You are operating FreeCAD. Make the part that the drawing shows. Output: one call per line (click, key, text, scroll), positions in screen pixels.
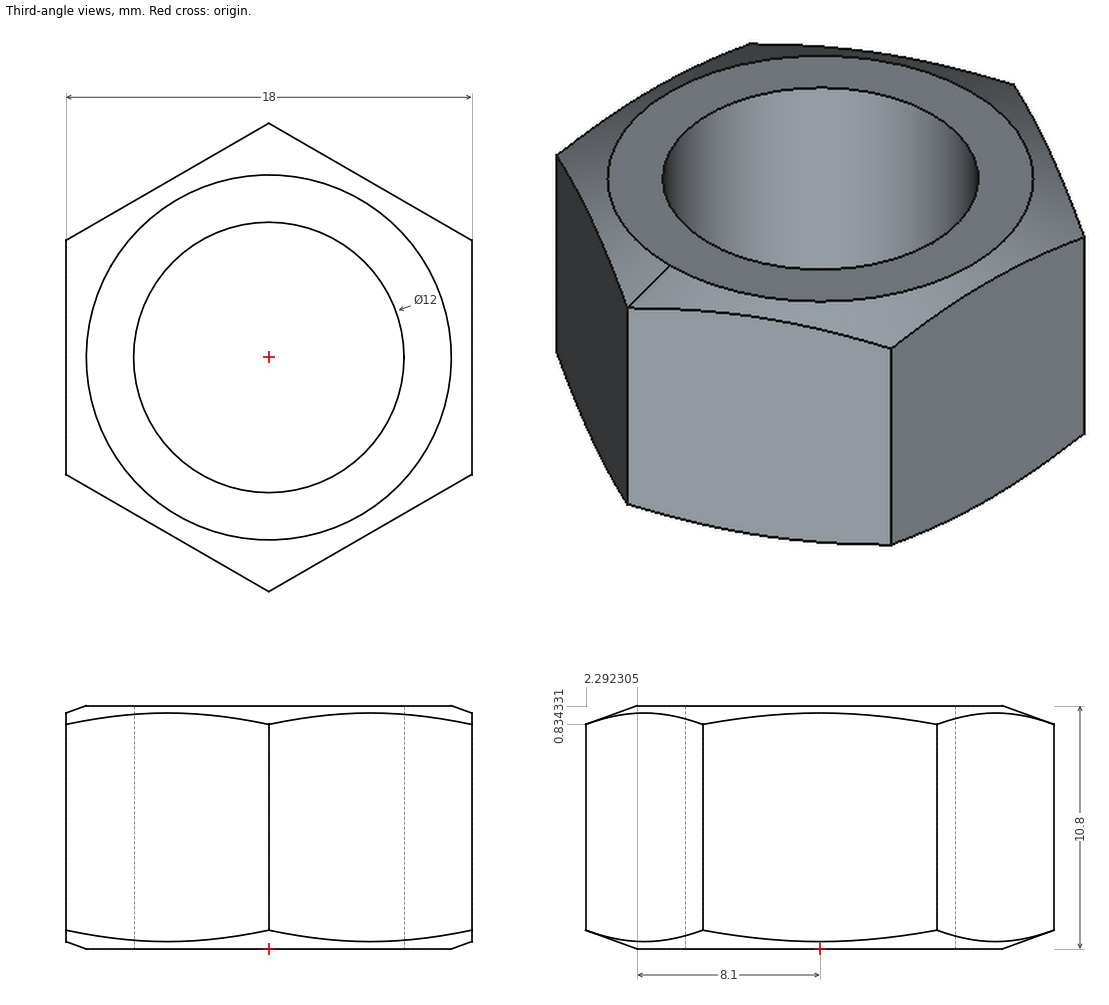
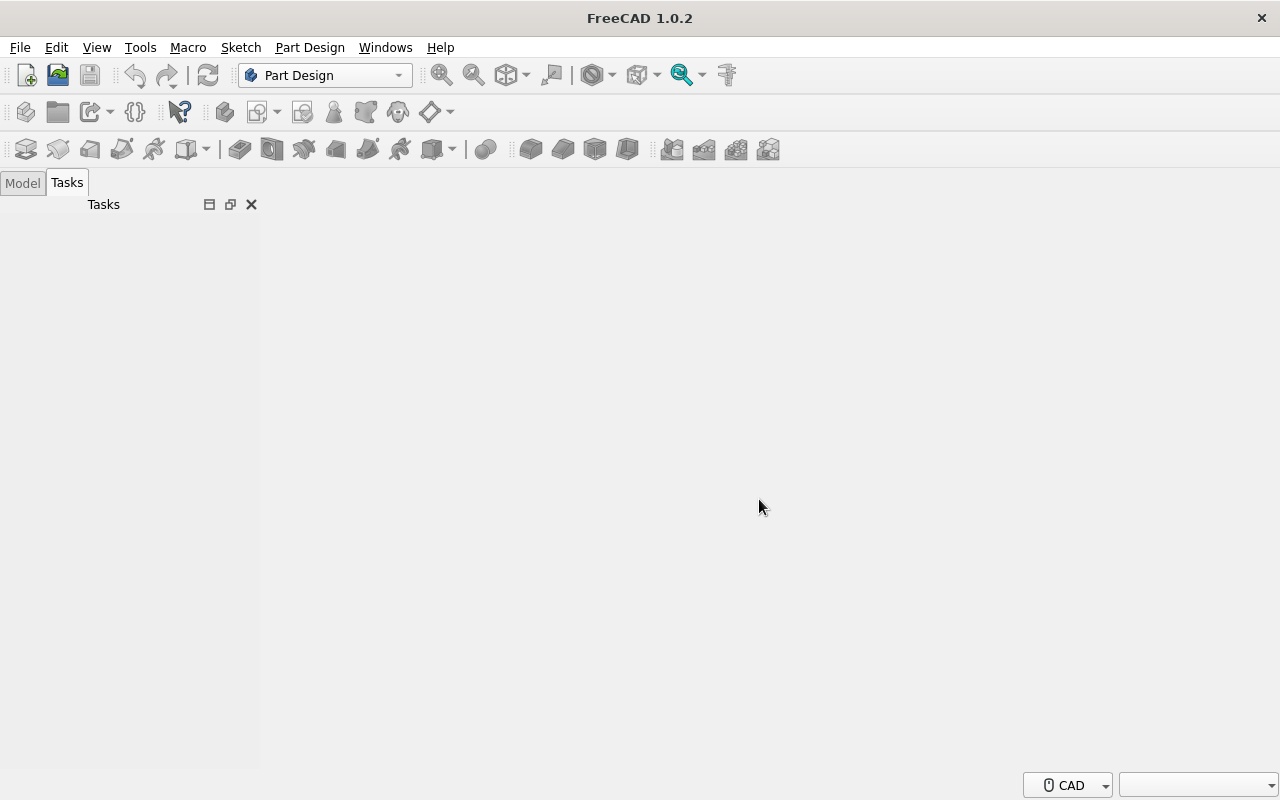
key(ctrl+n)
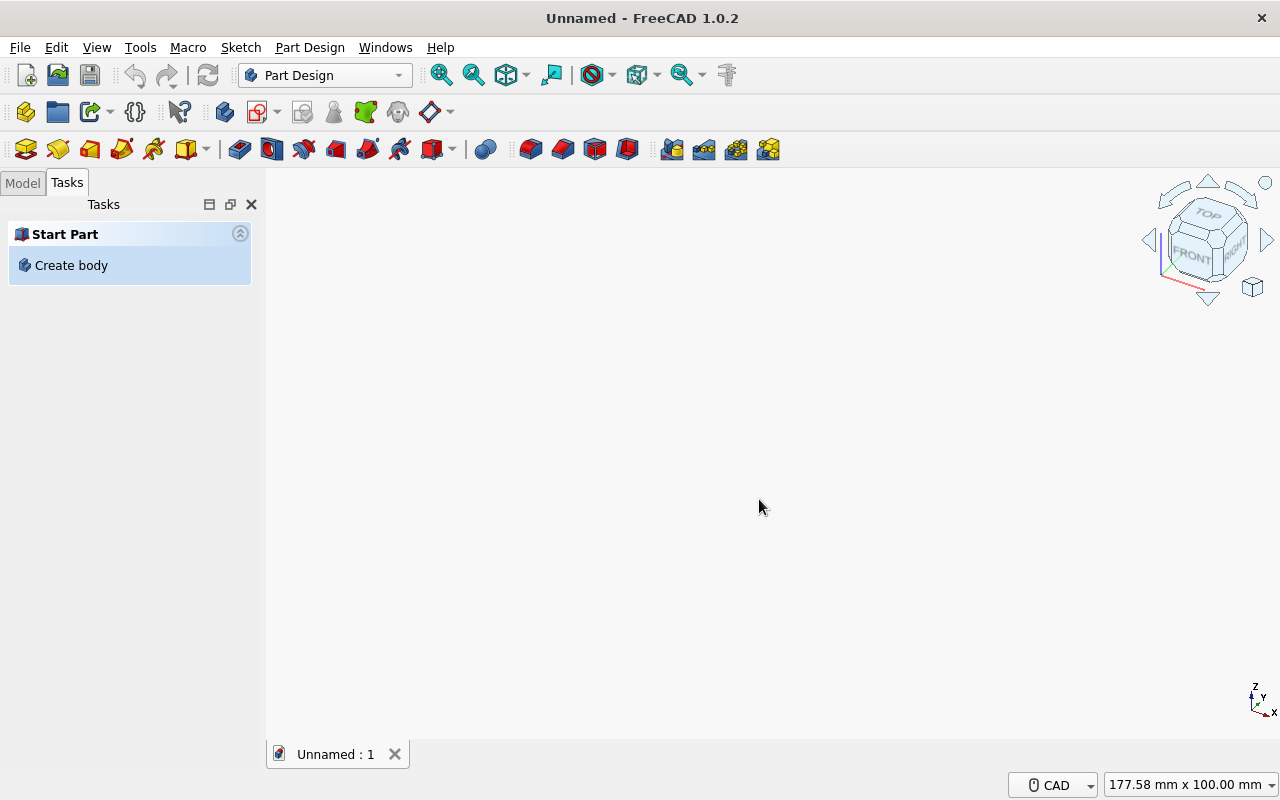
click(258, 112)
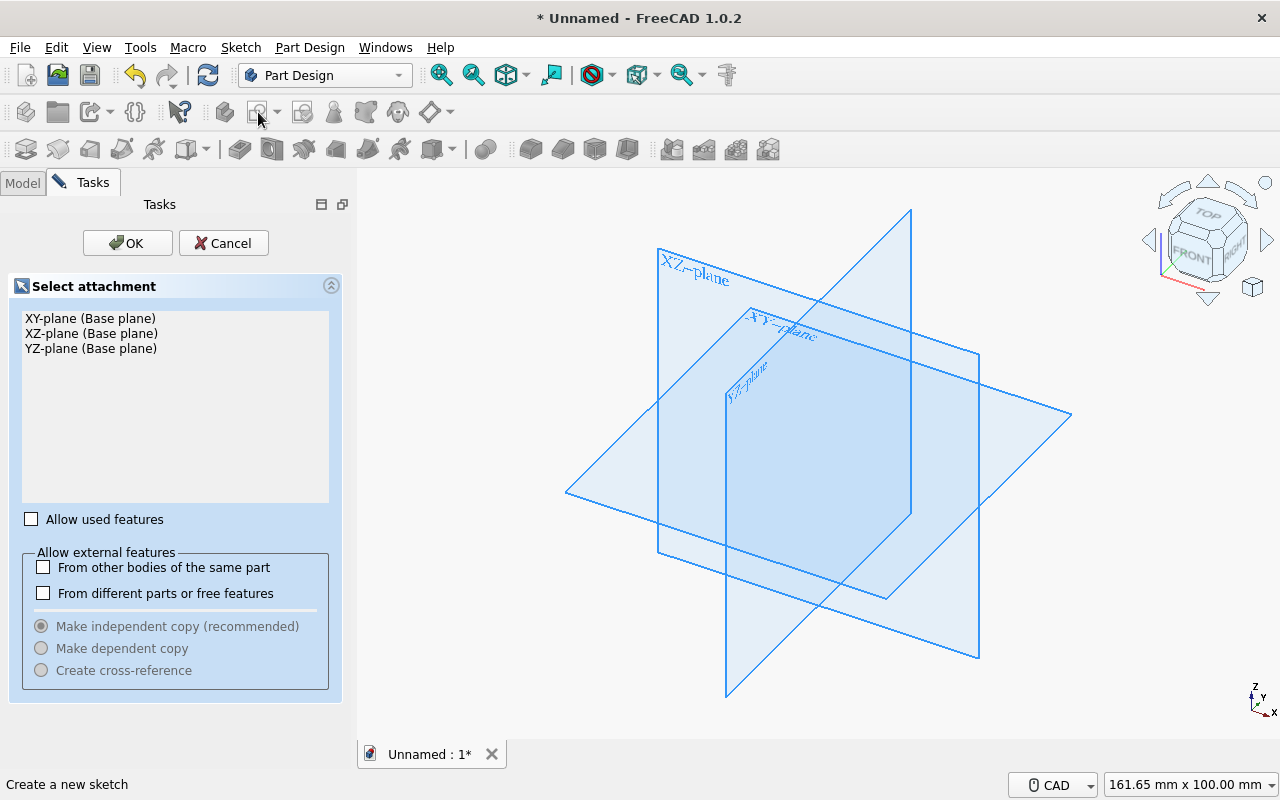
click(82, 318)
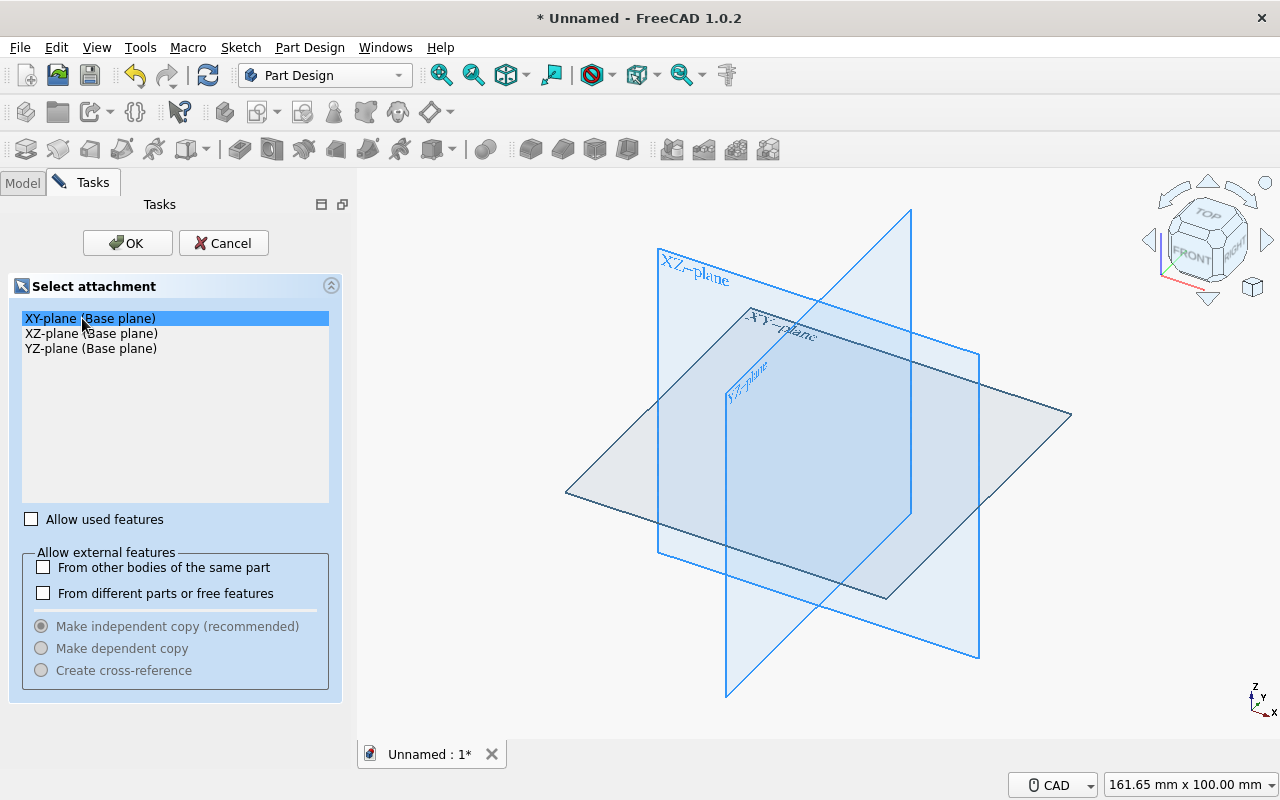
click(128, 243)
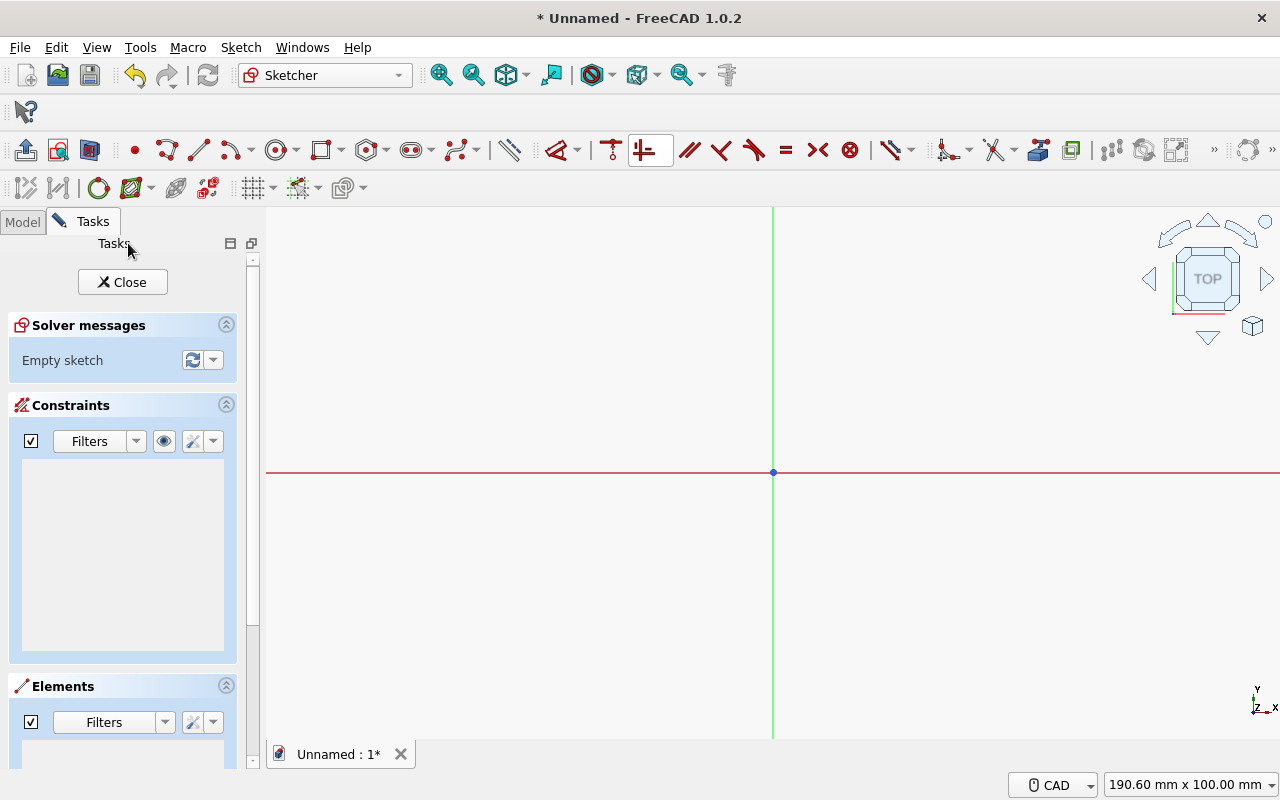
scroll(803, 473, up, 6)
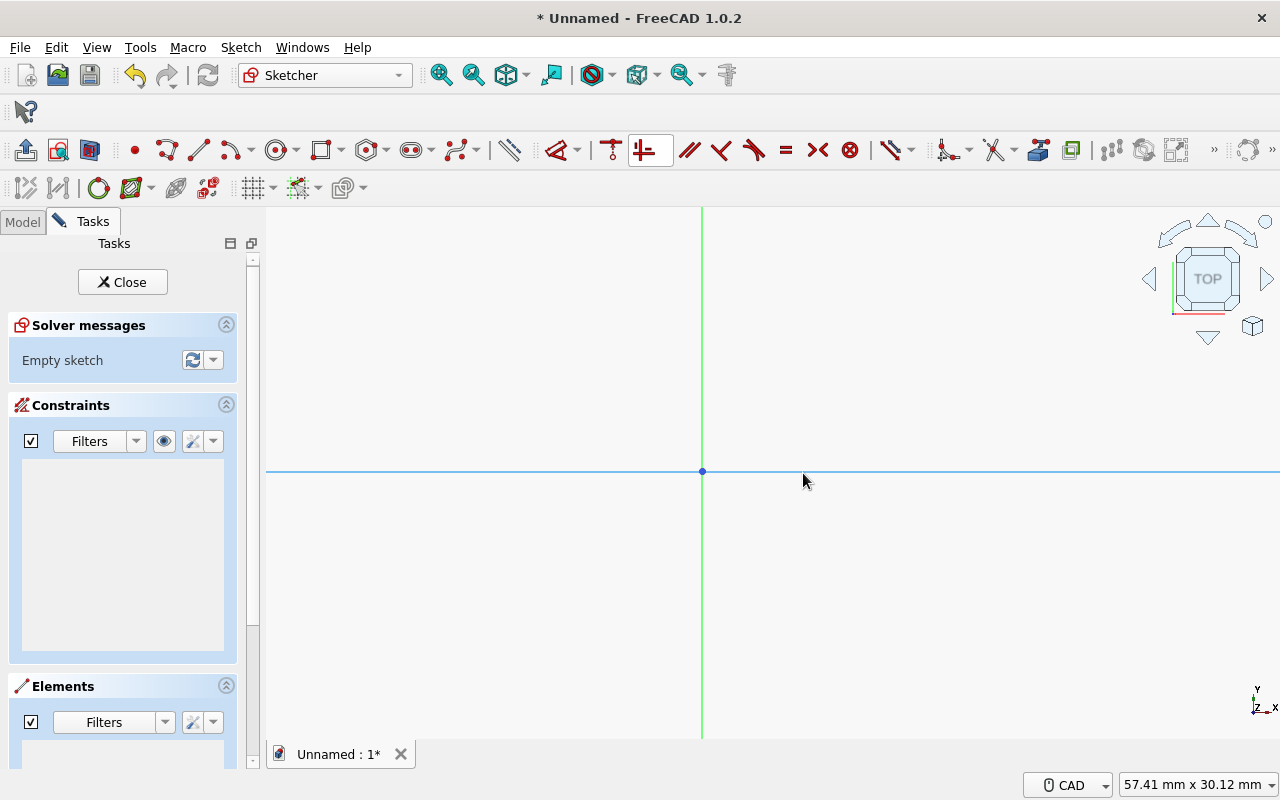
click(366, 150)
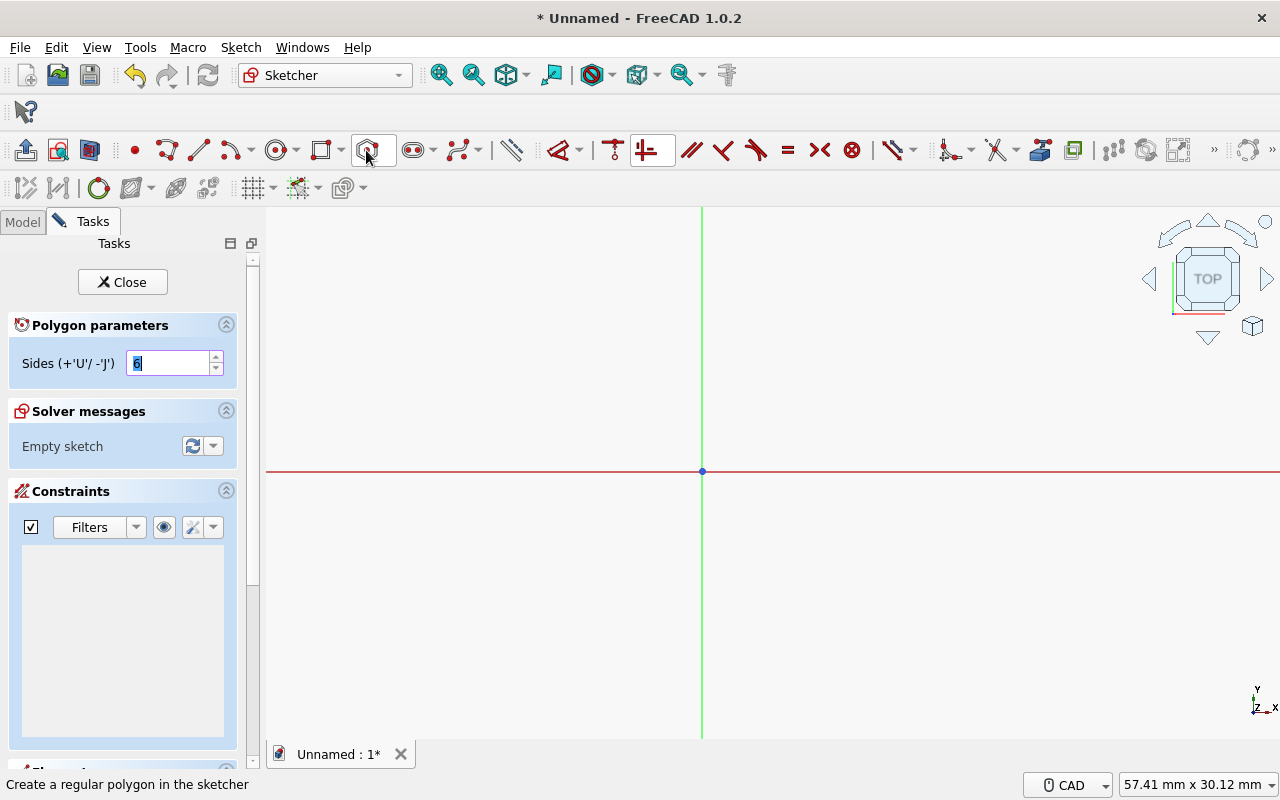
click(702, 472)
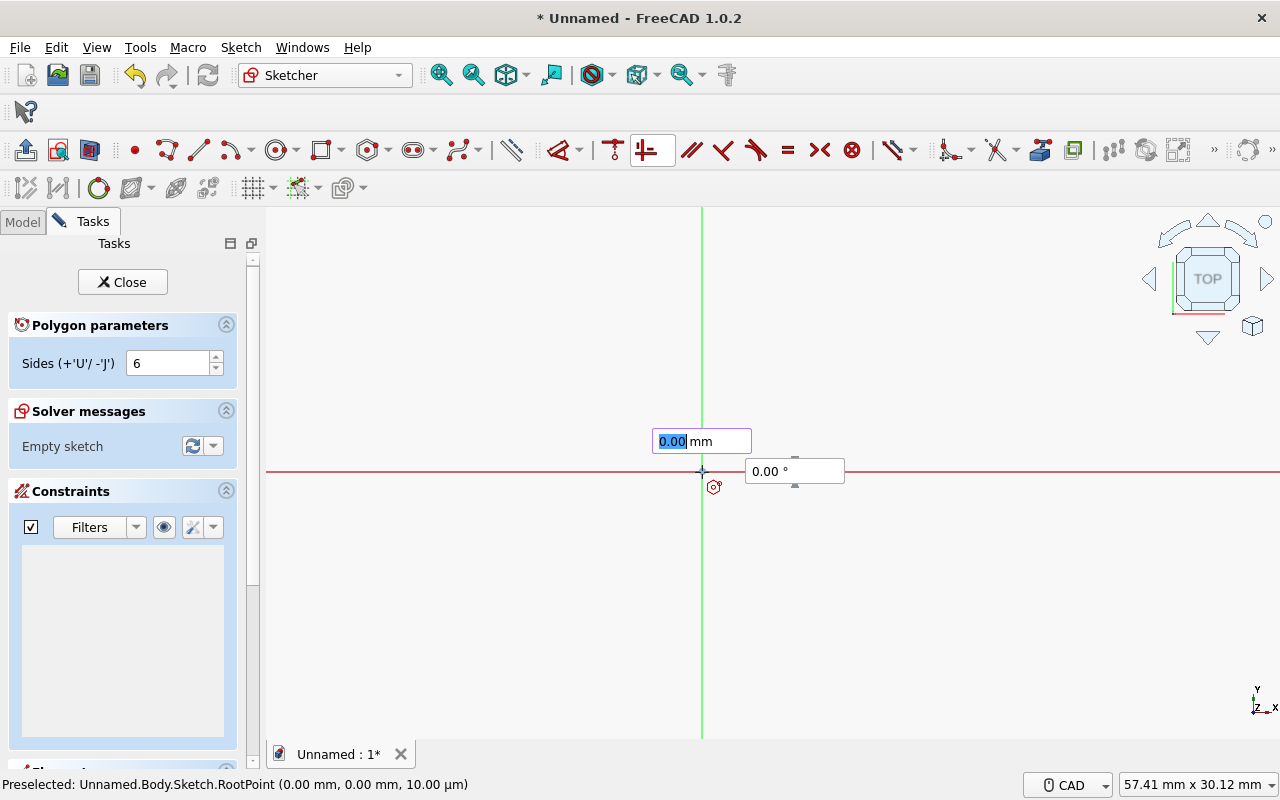
click(702, 288)
right_click(702, 288)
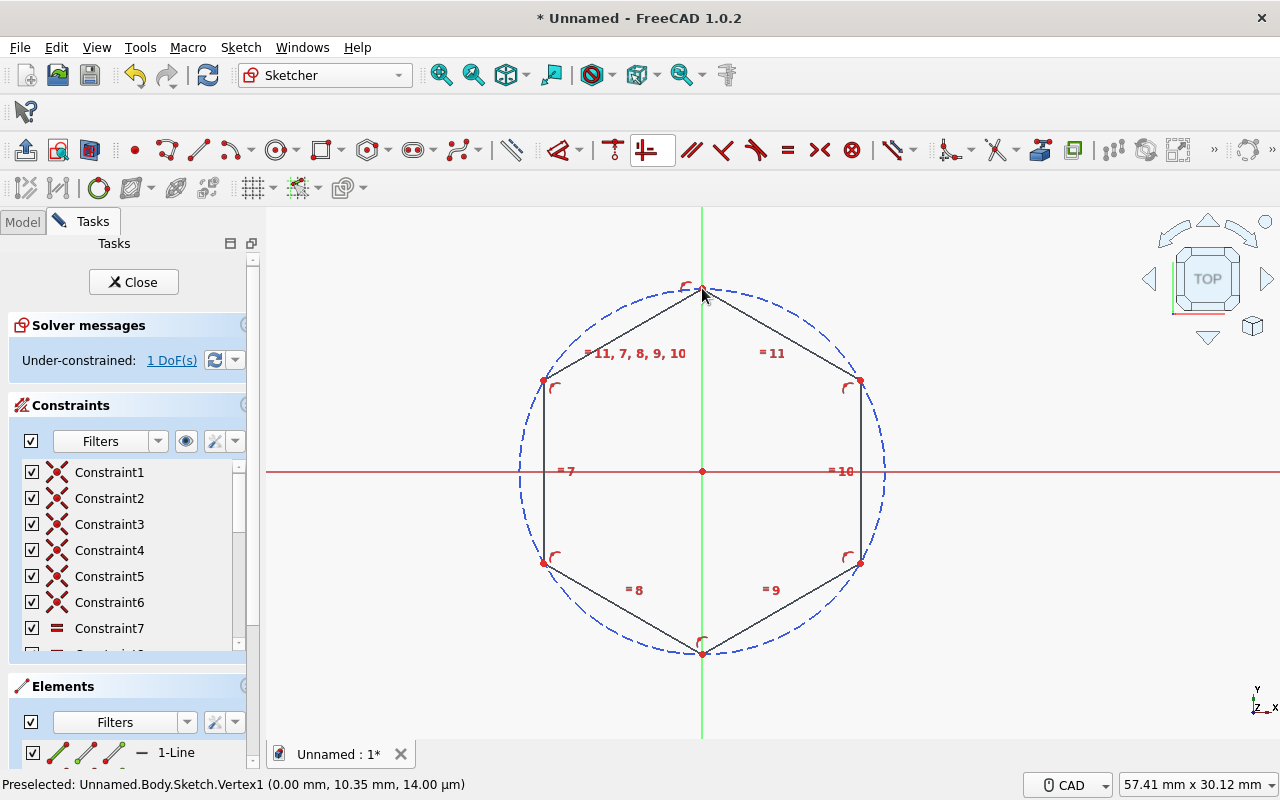
click(558, 150)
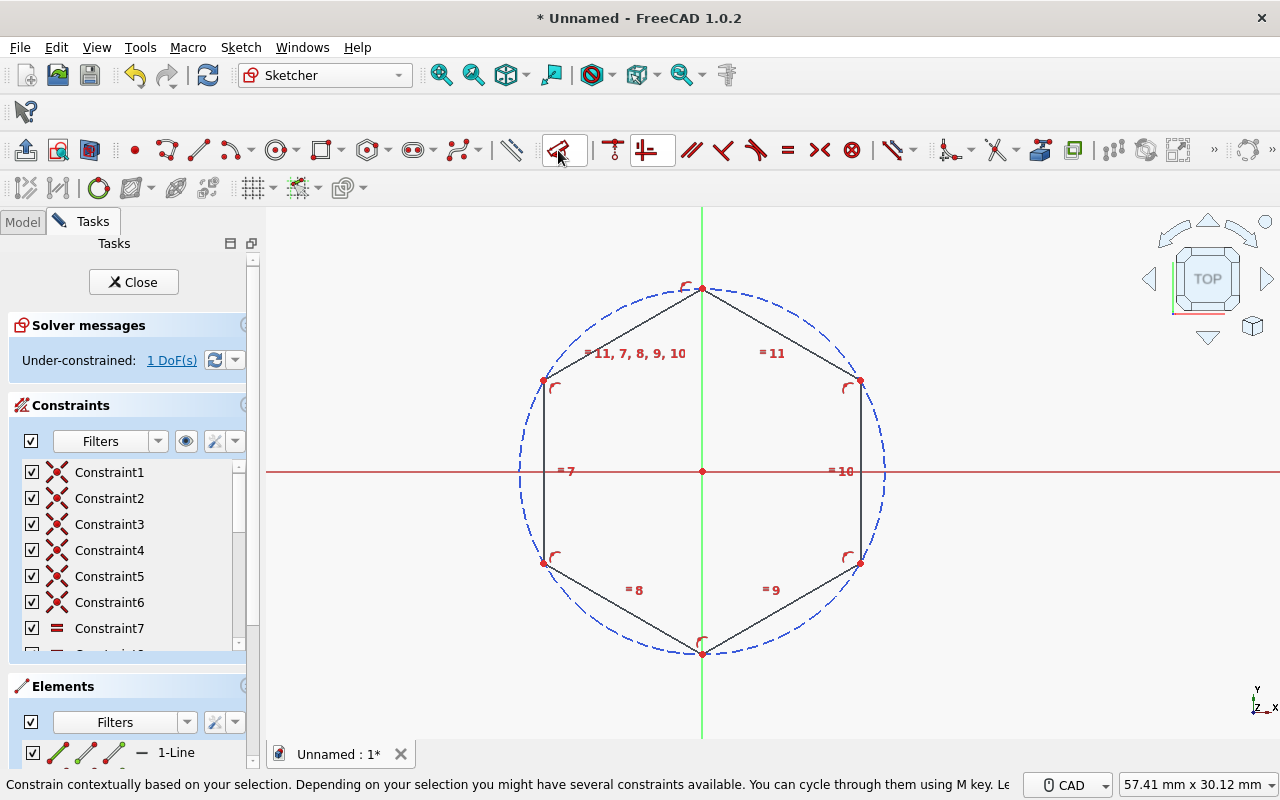
click(544, 380)